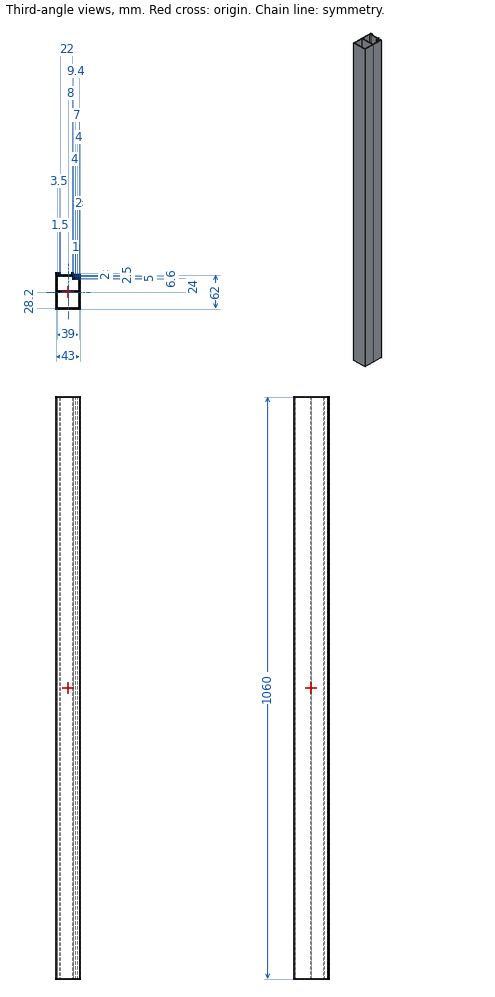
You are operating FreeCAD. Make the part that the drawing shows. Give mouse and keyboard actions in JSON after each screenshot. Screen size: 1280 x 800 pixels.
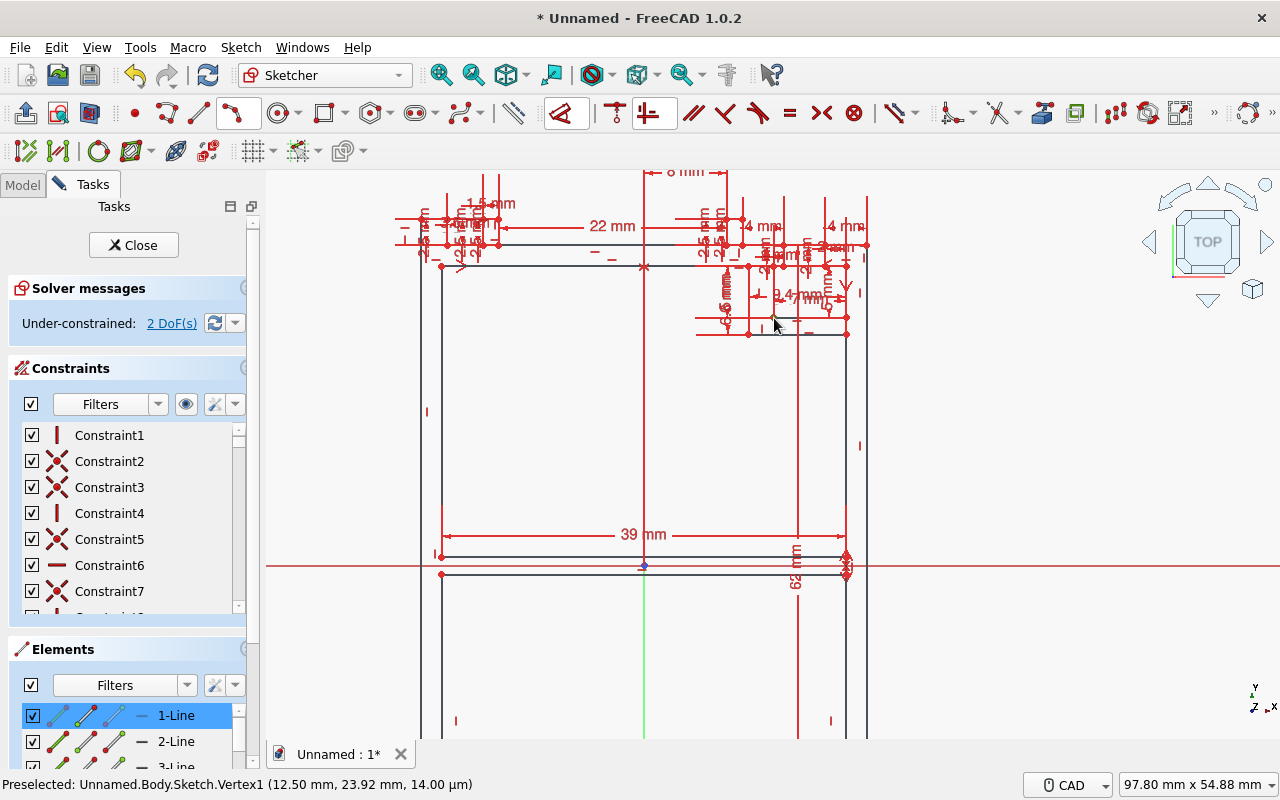
{"action": "key", "text": "i"}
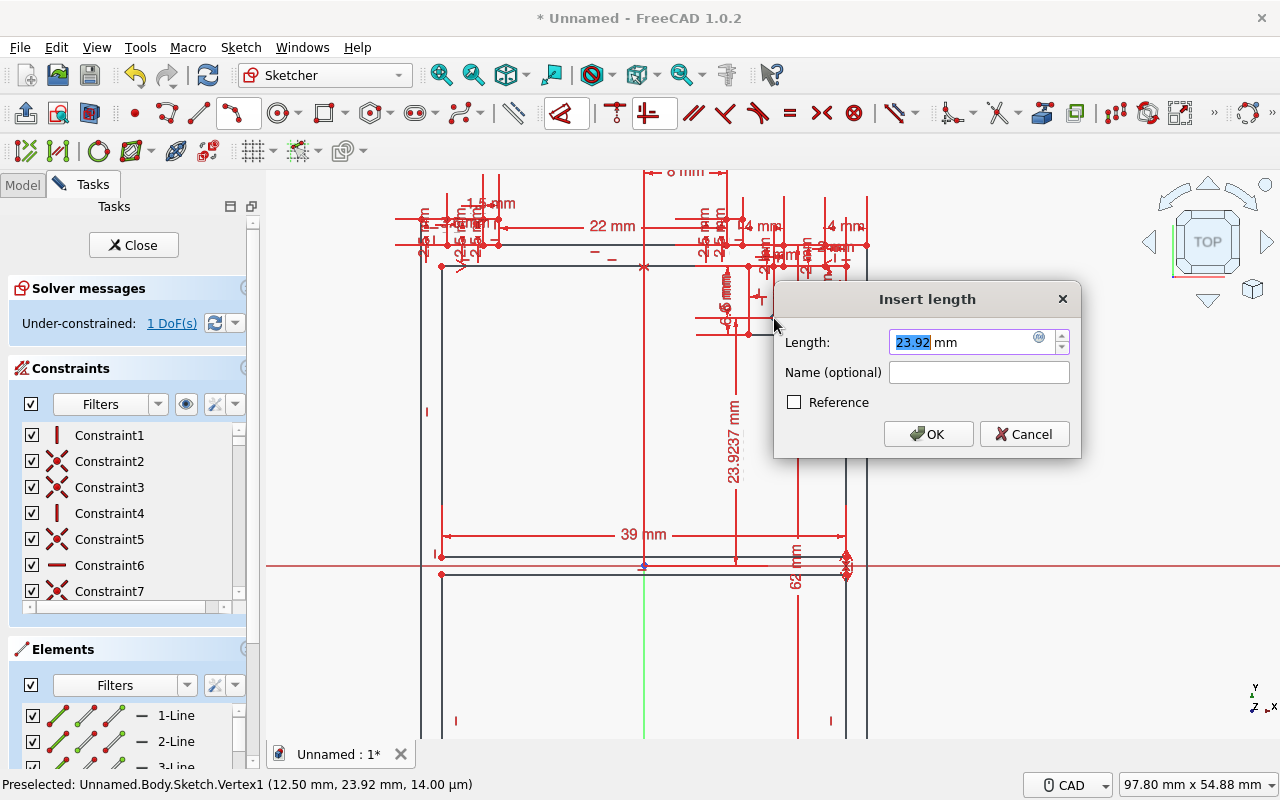
{"action": "type", "text": "24"}
{"action": "key", "text": "Return"}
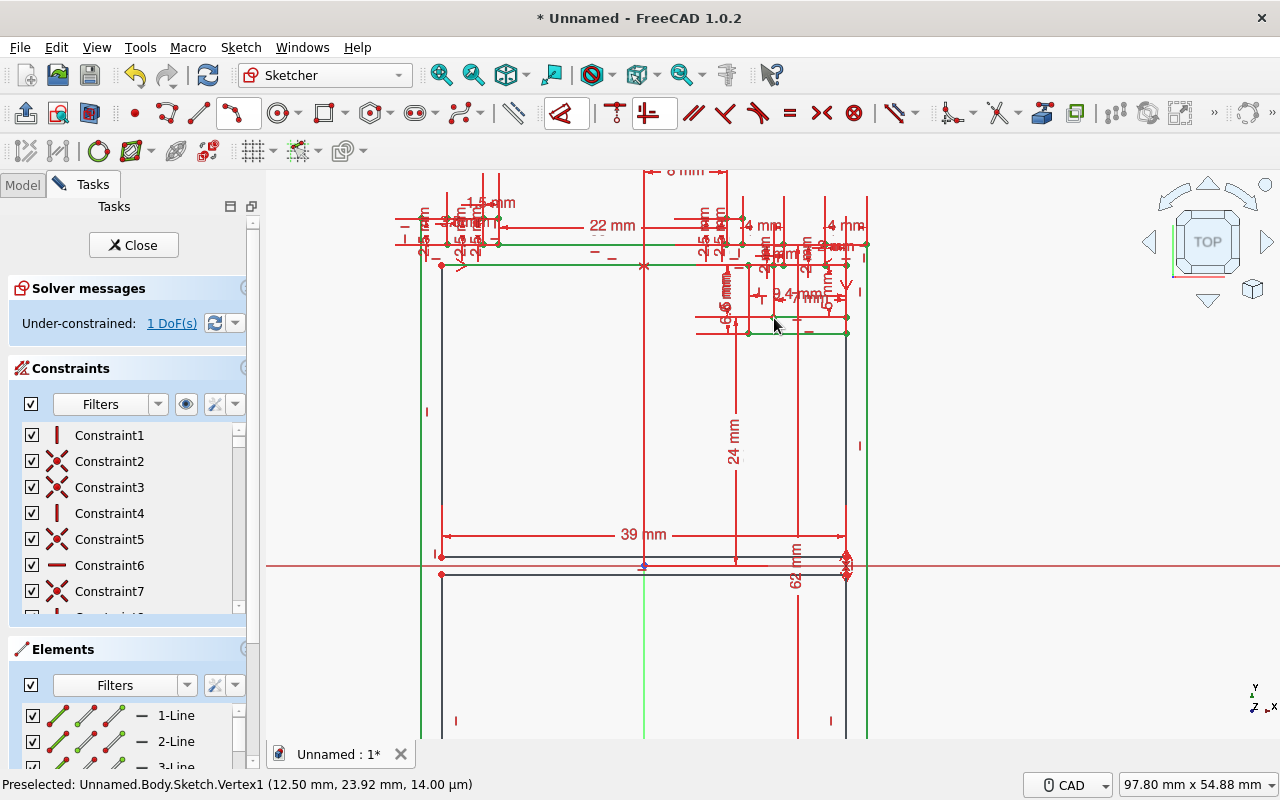
{"action": "left_click", "coordinate": [442, 662]}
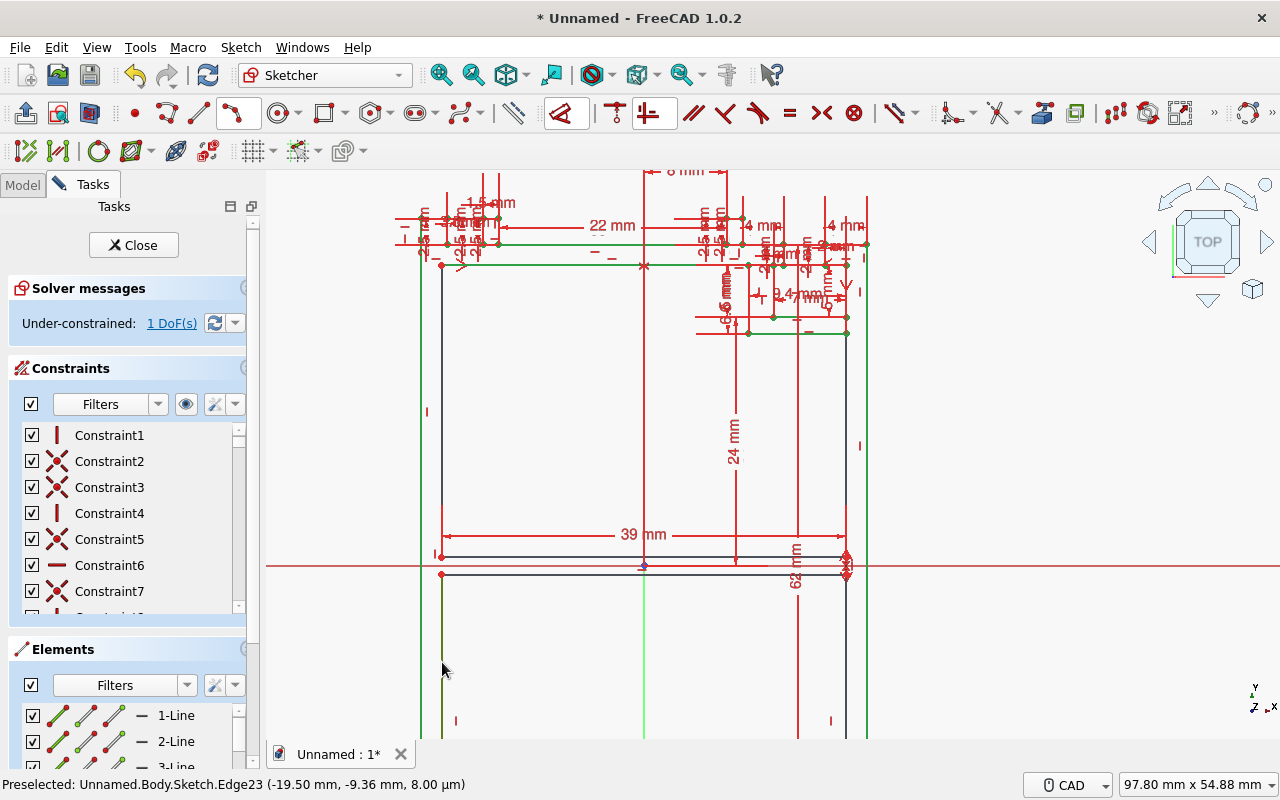
{"action": "left_click", "coordinate": [584, 114]}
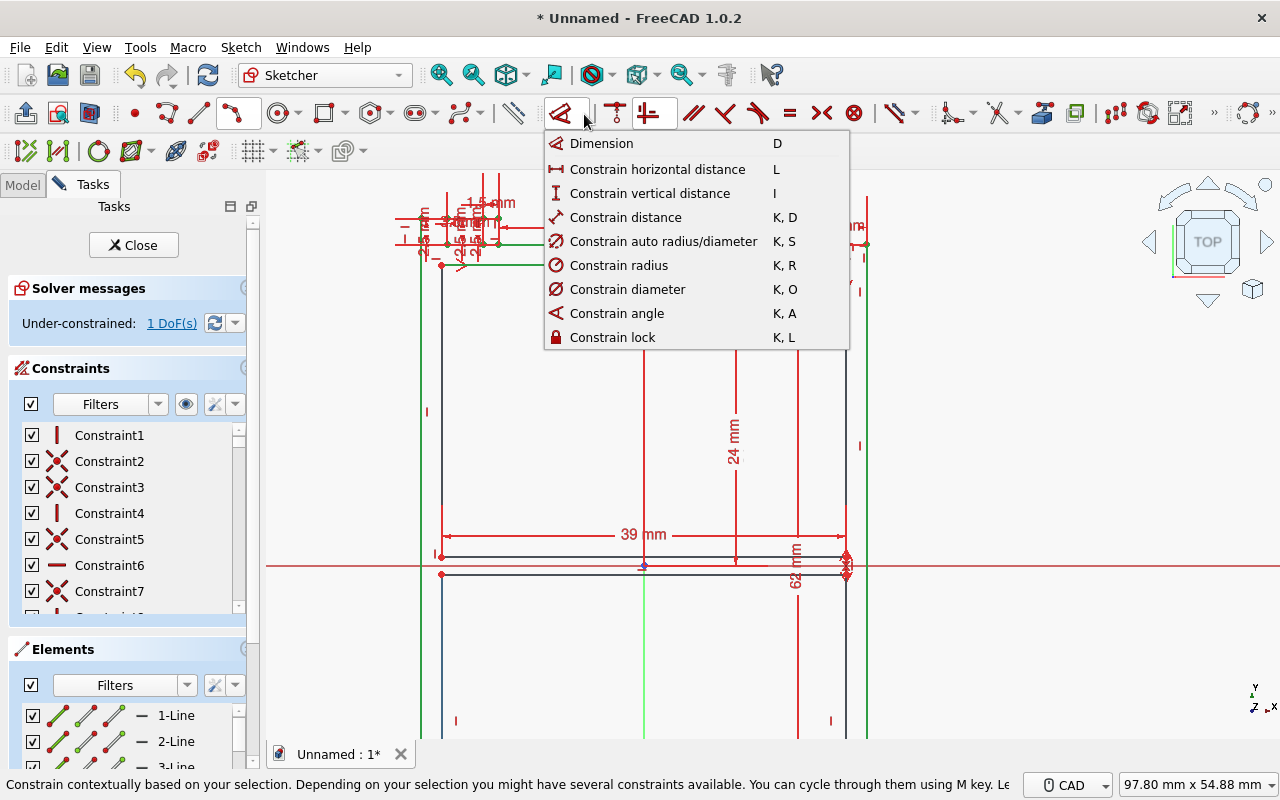
{"action": "left_click", "coordinate": [697, 193]}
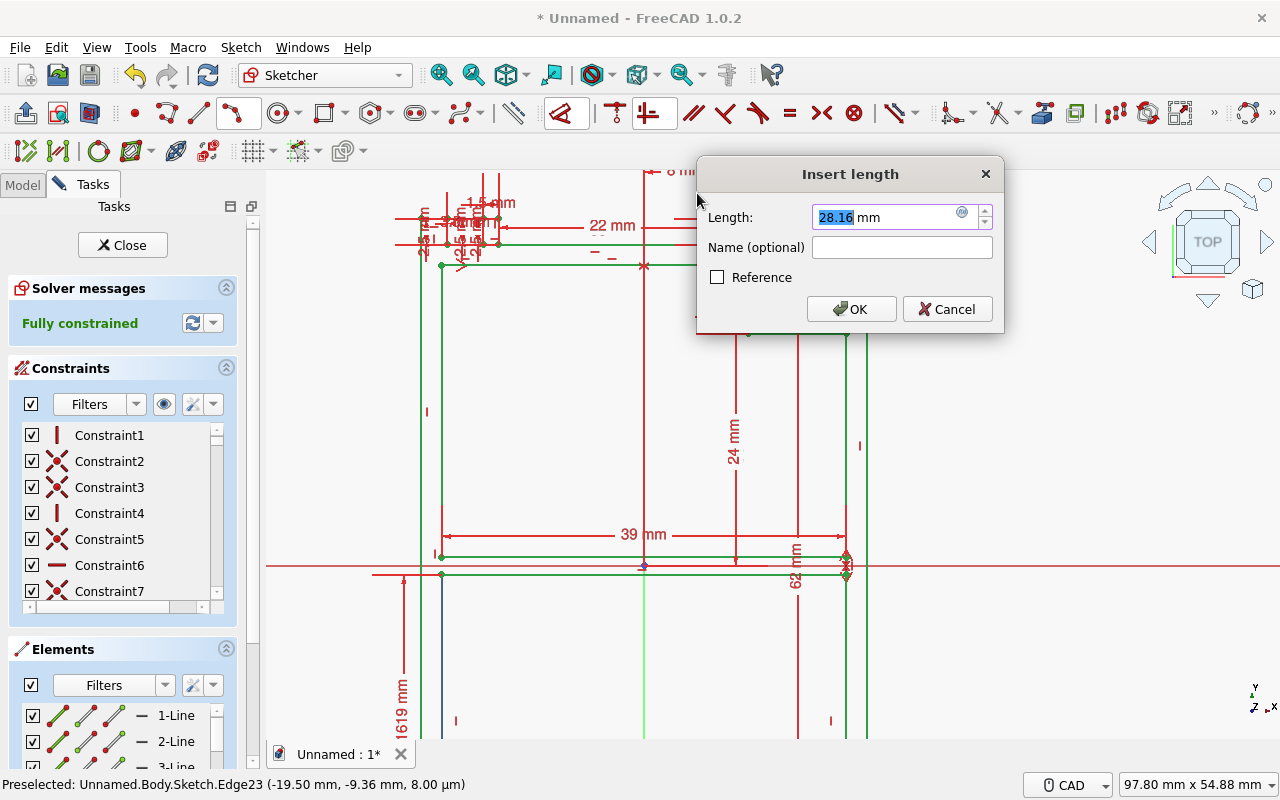
{"action": "type", "text": "28.2"}
{"action": "key", "text": "Return"}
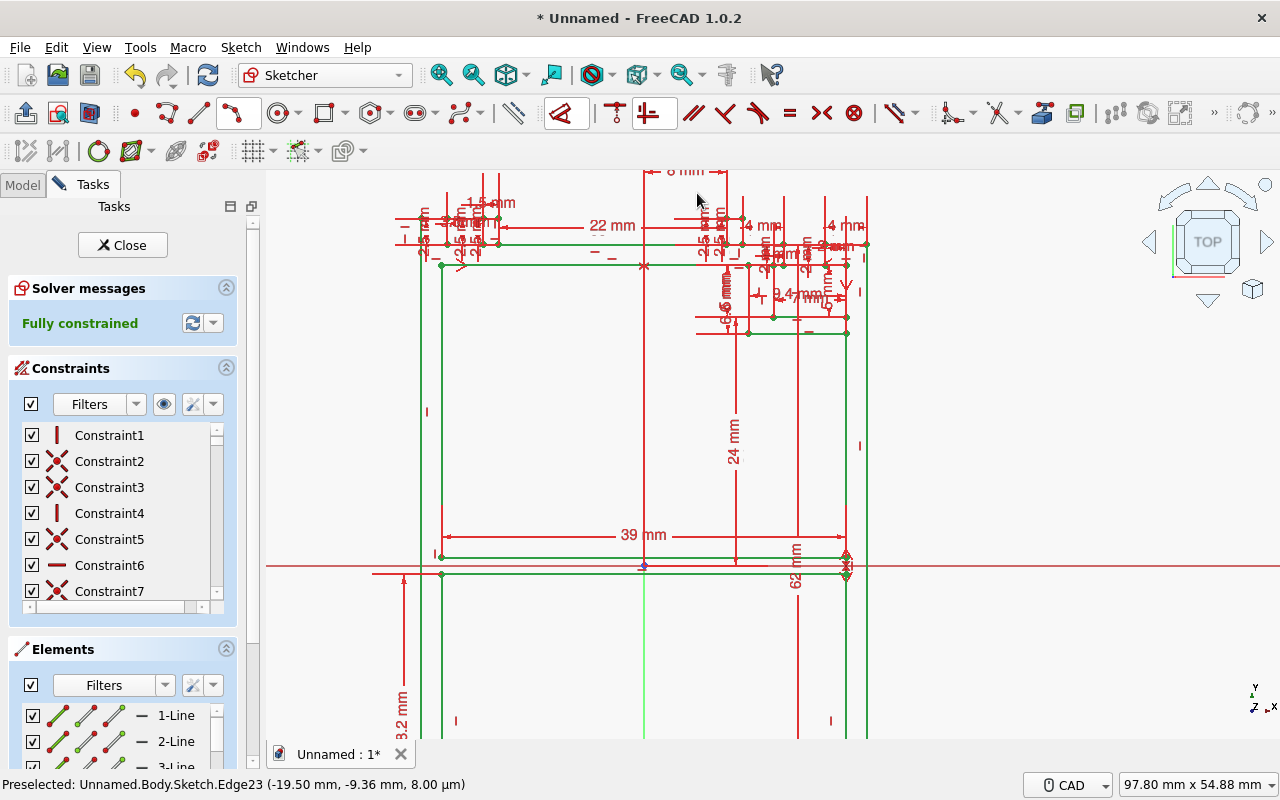
{"action": "left_click", "coordinate": [123, 245]}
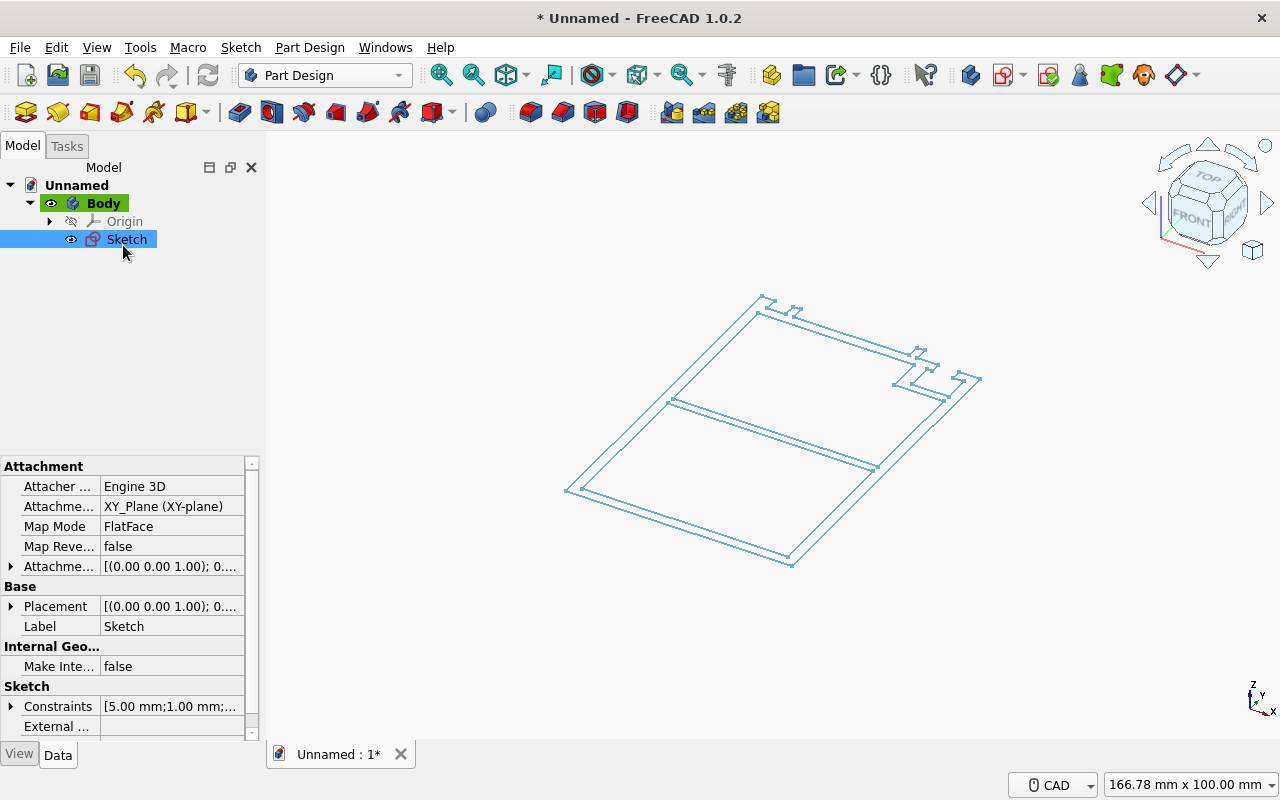
{"action": "left_click", "coordinate": [26, 112]}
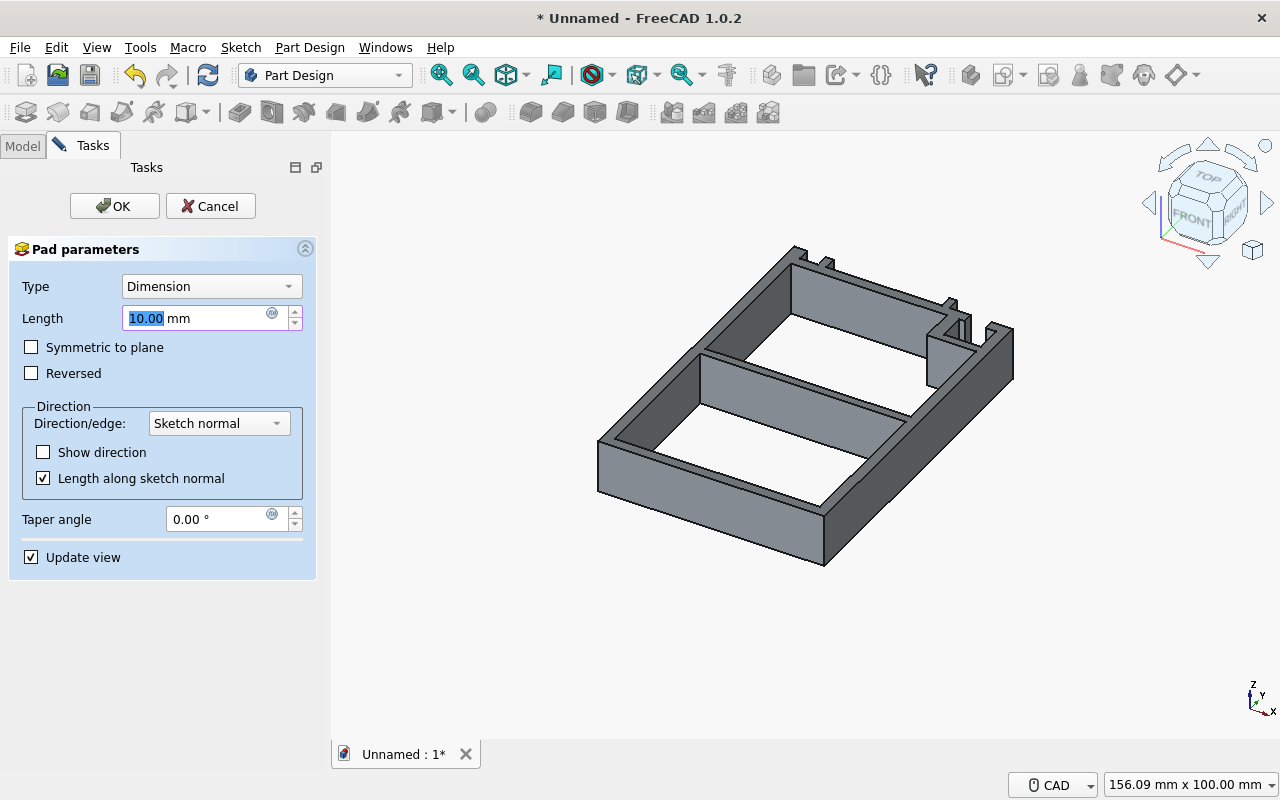
{"action": "type", "text": "1060"}
{"action": "key", "text": "Tab"}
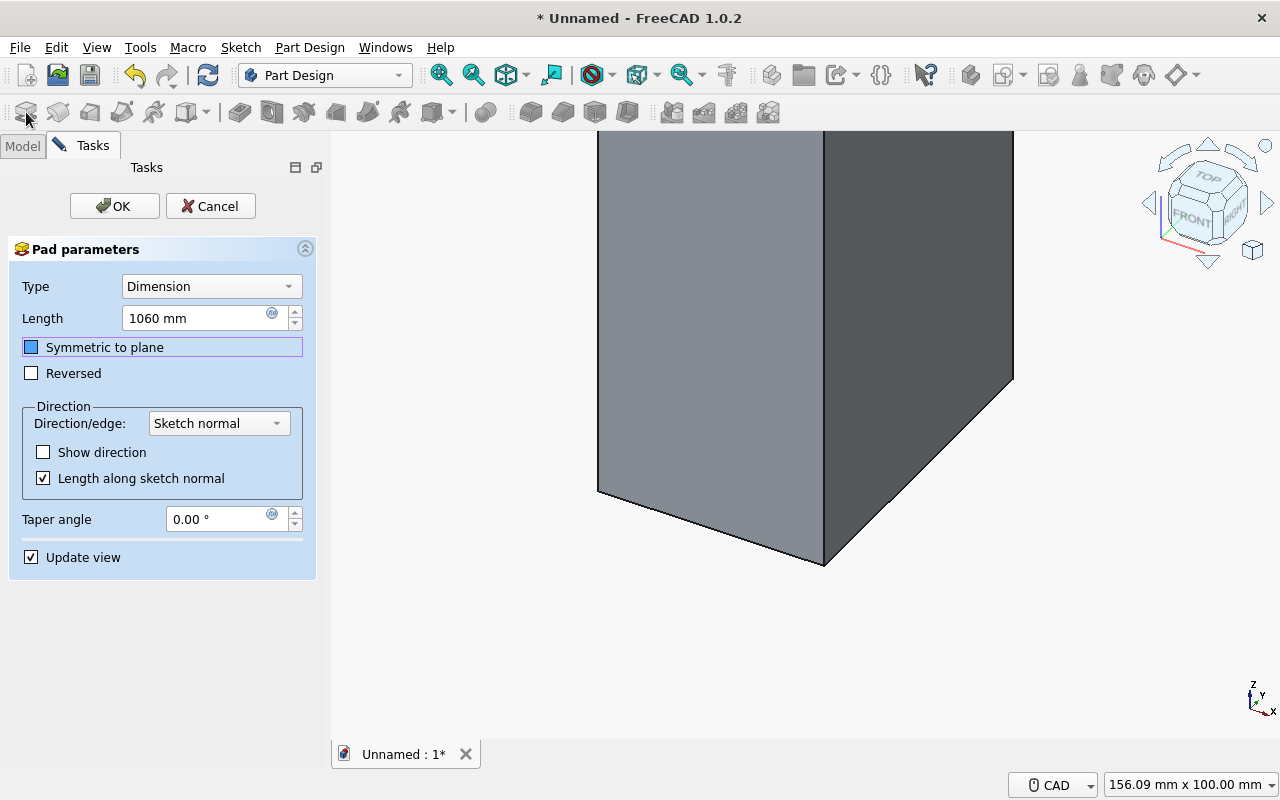
{"action": "left_click", "coordinate": [30, 347]}